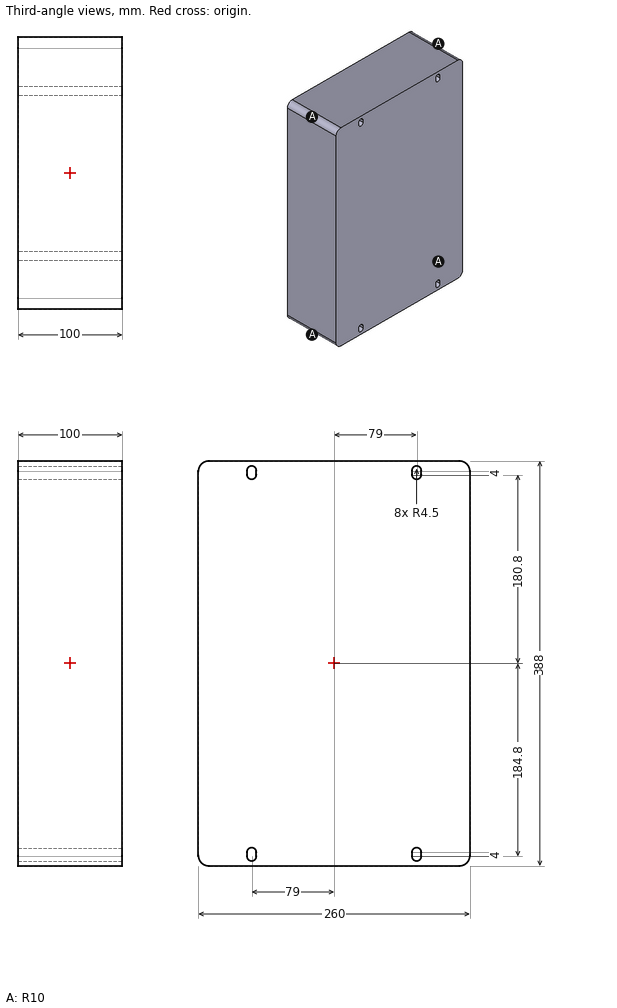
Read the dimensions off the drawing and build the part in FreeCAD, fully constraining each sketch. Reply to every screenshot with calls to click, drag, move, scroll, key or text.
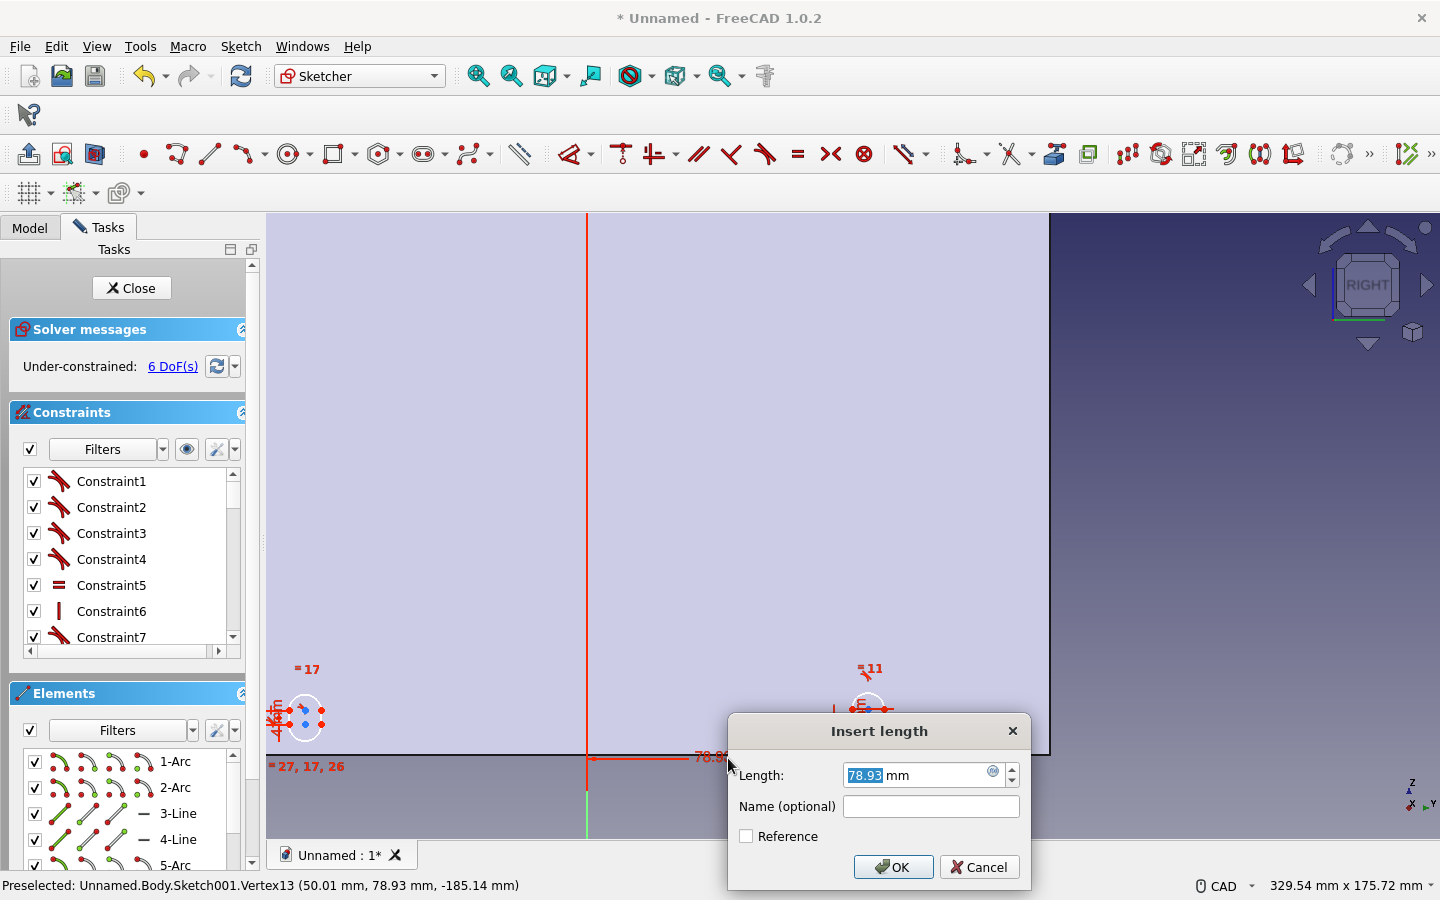
text(79)
key(Return)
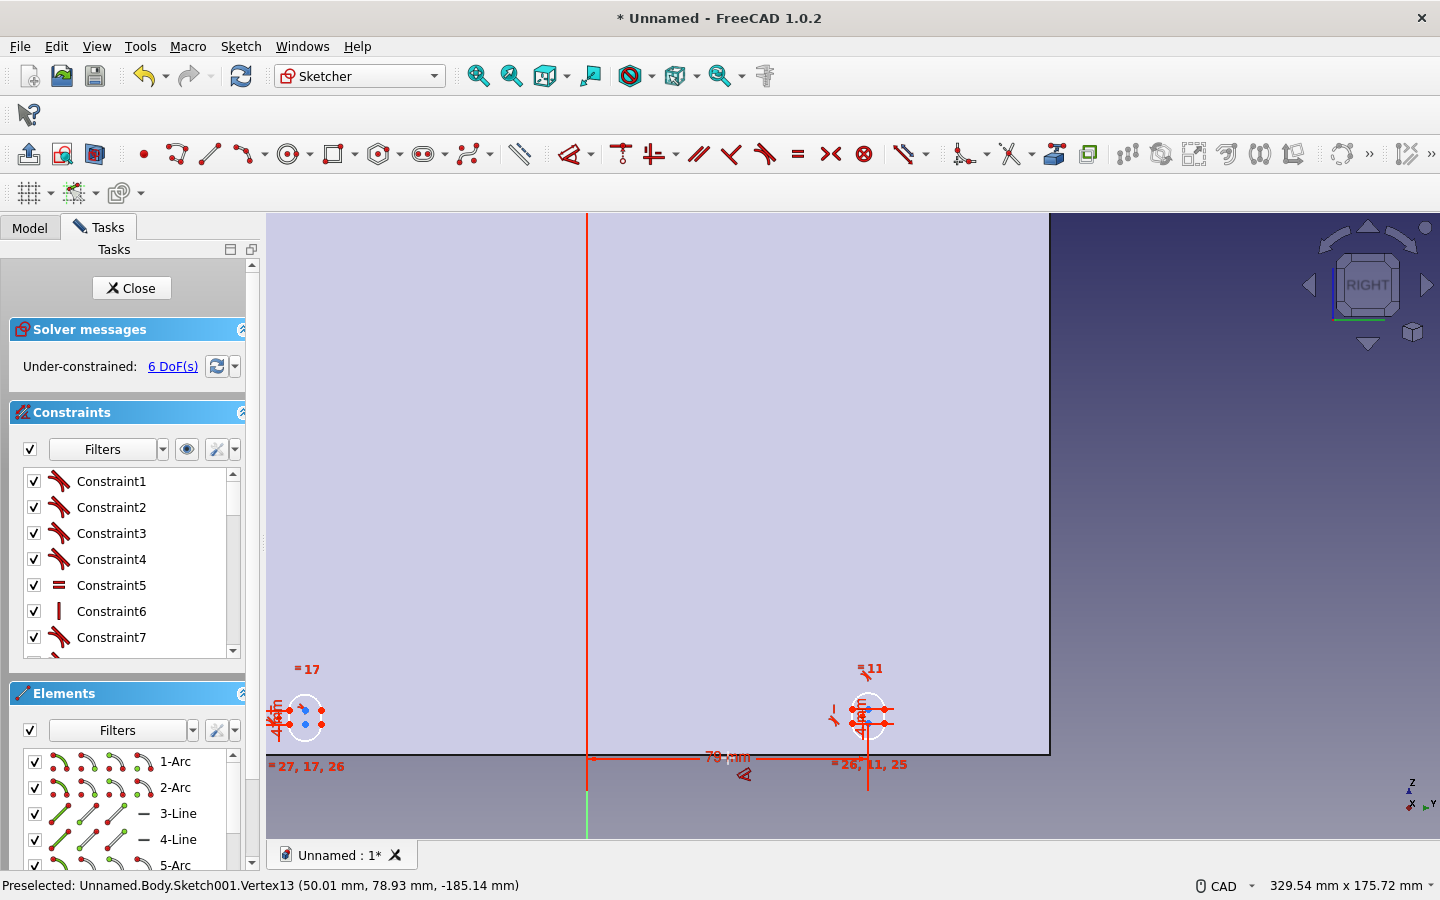
click(305, 725)
click(446, 759)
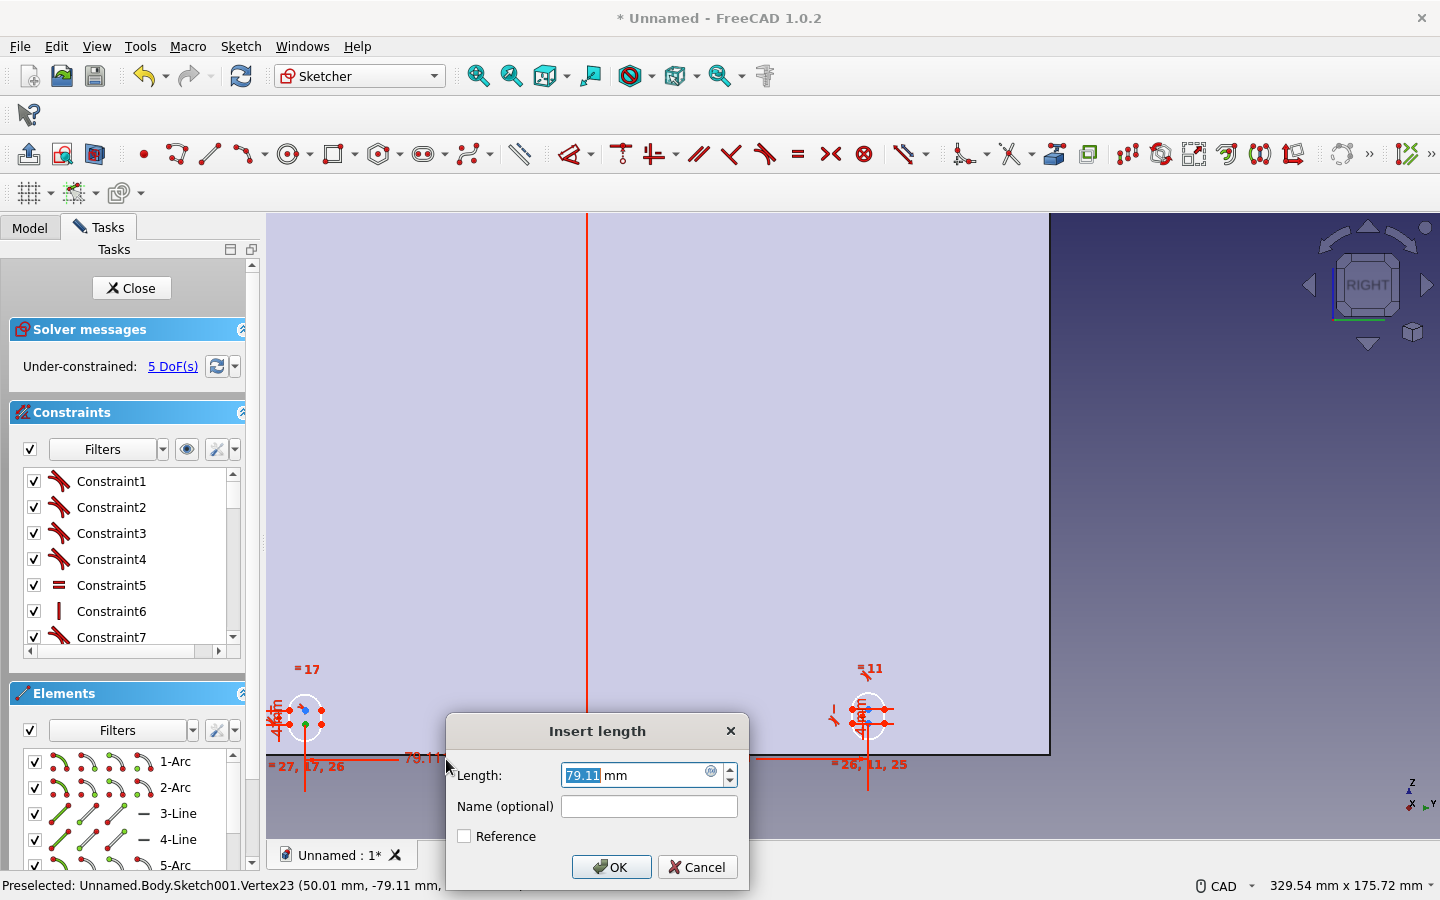
text(79)
key(Return)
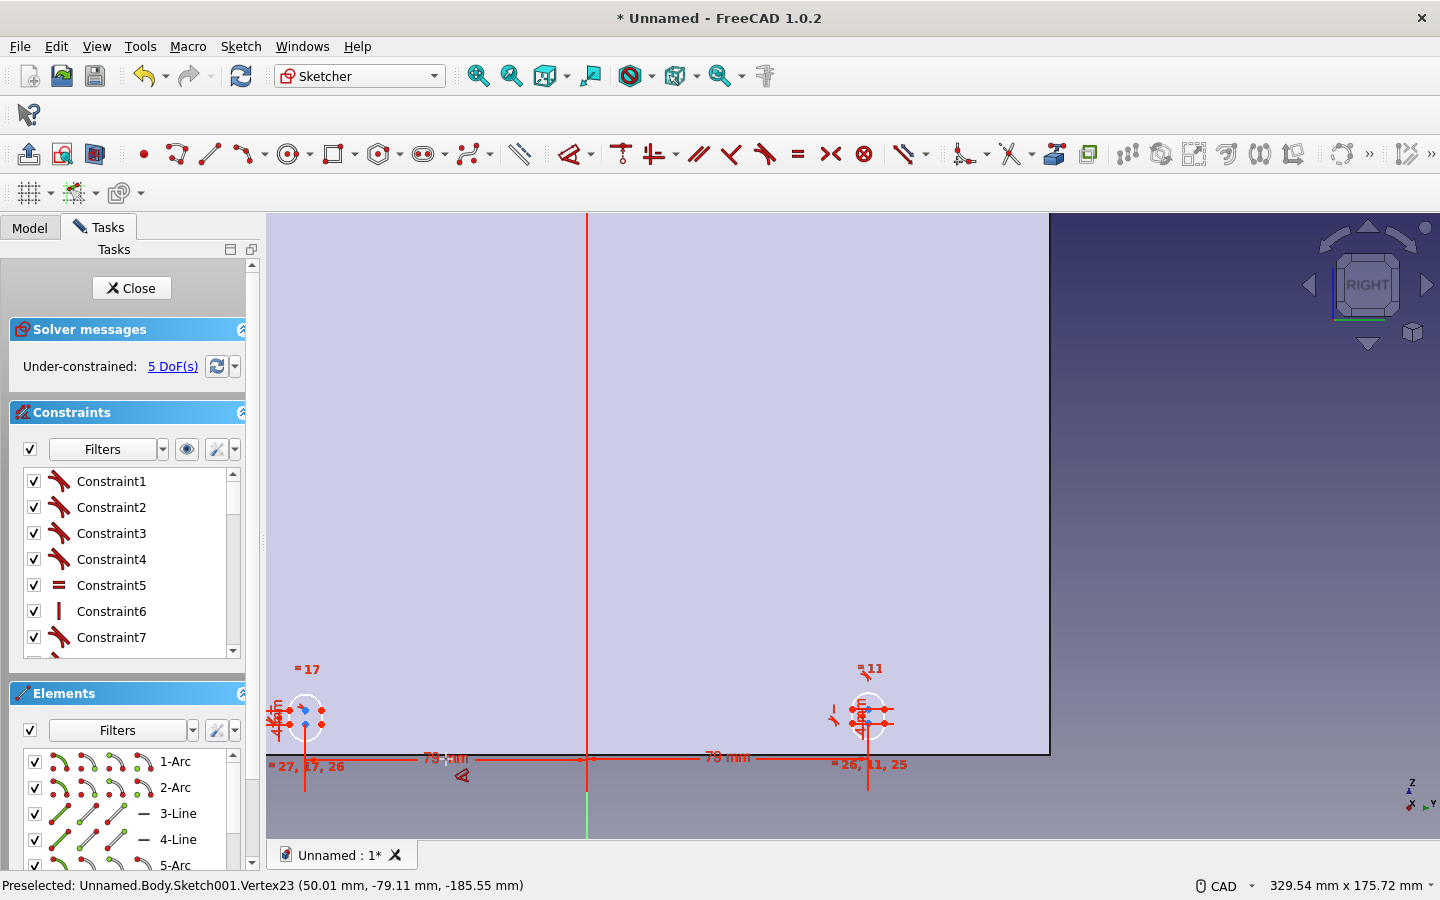
scroll(870, 725, down, 6)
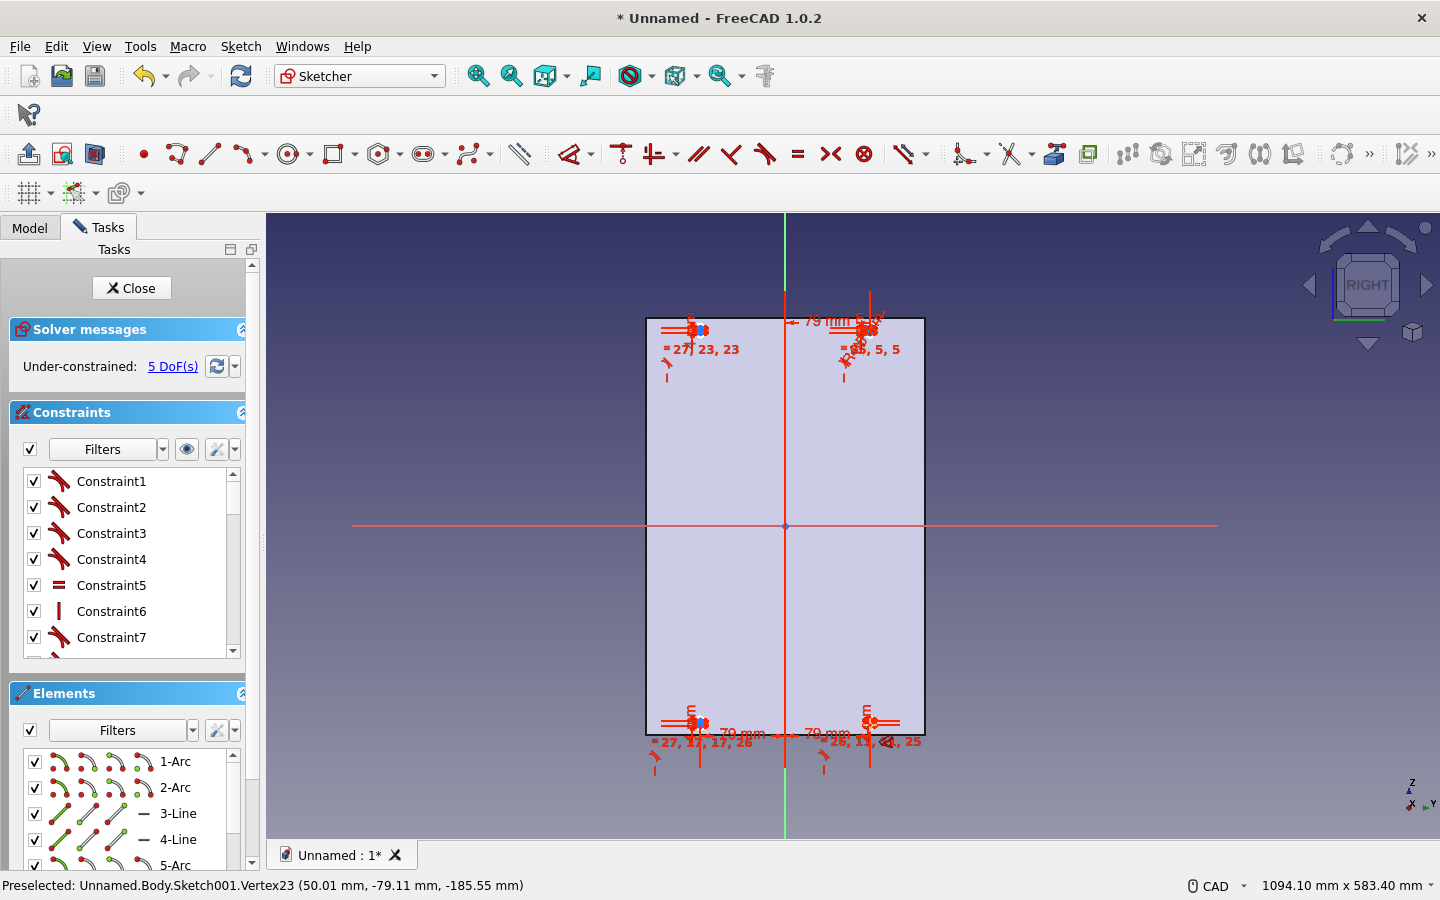
scroll(700, 333, up, 6)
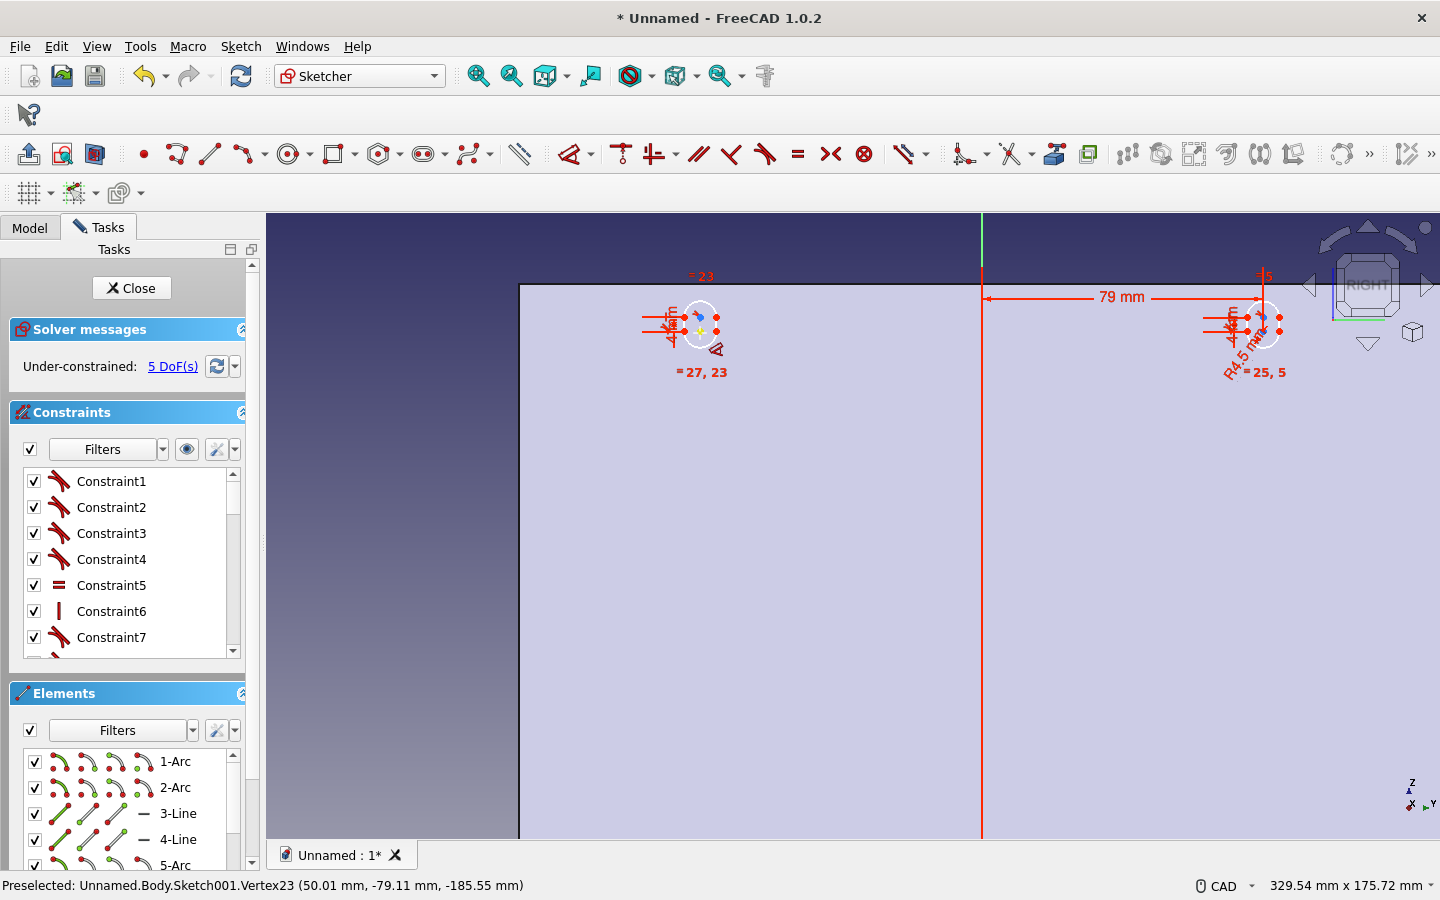
click(700, 332)
click(841, 298)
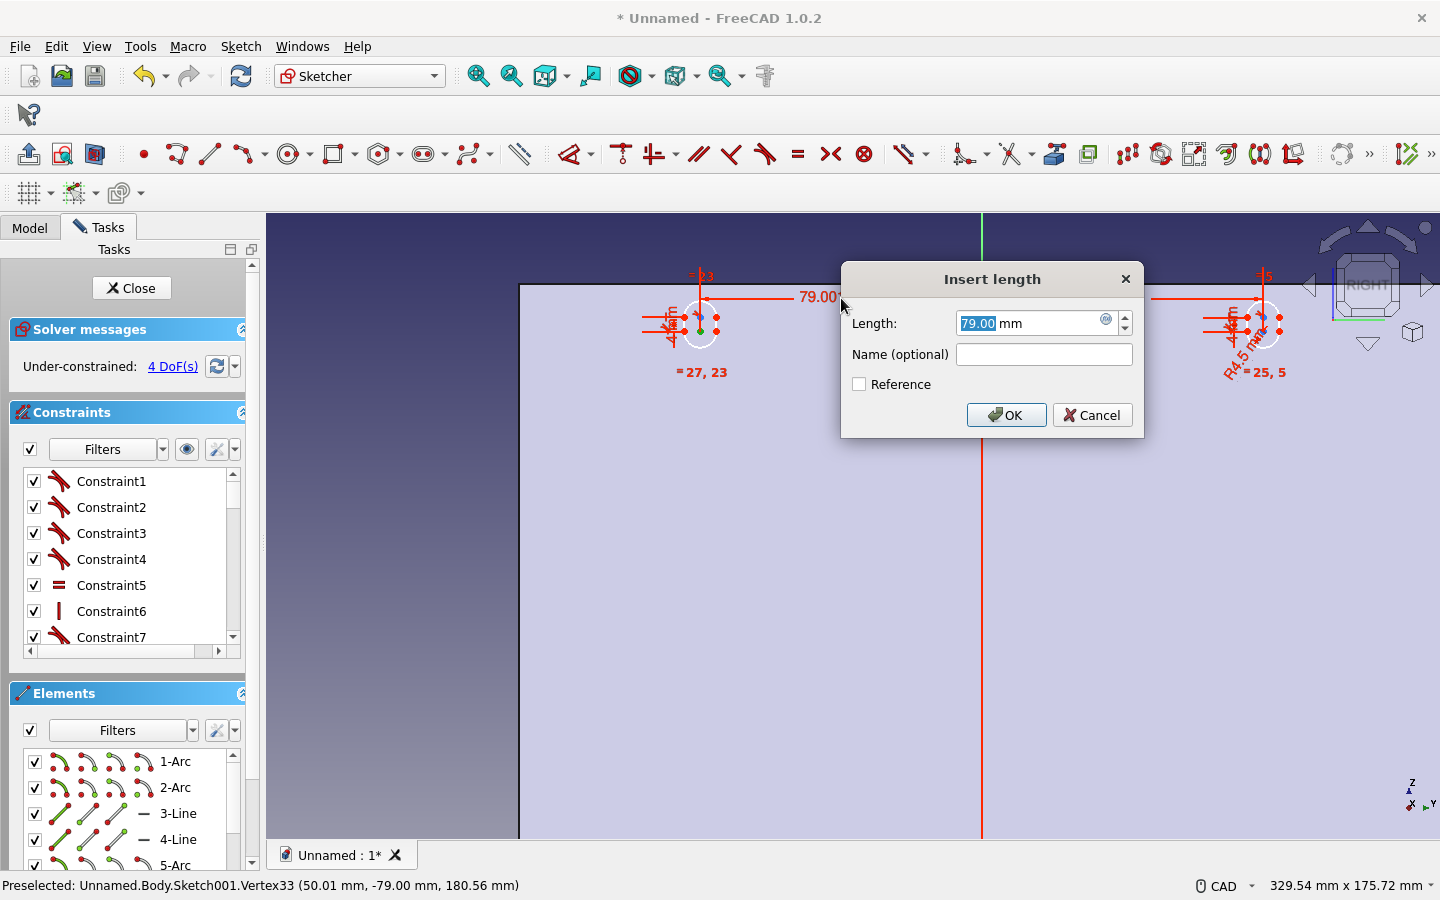
text(79)
key(Return)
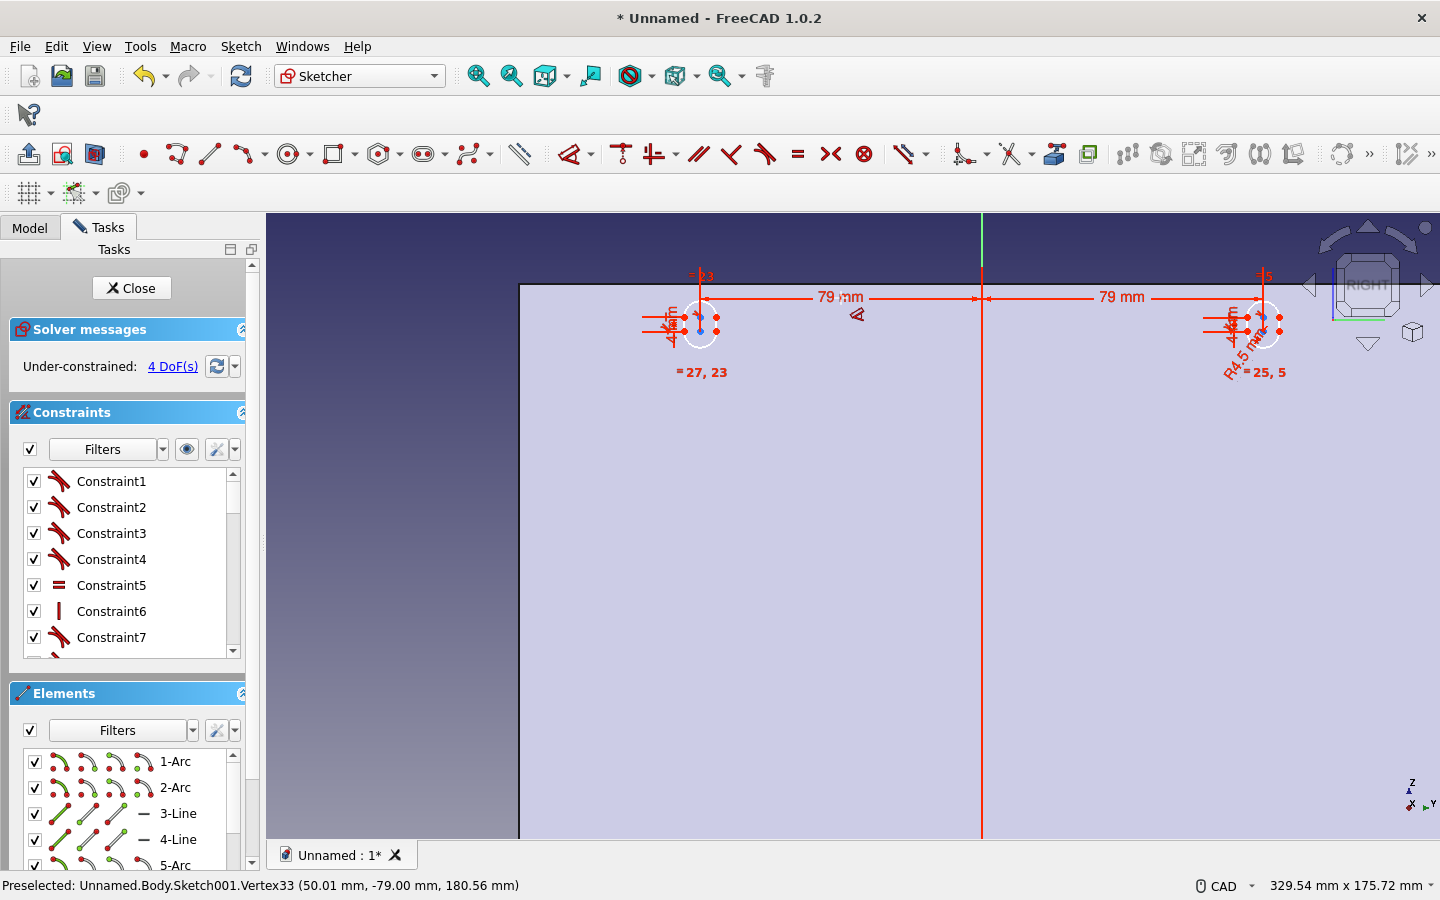
click(1247, 332)
click(948, 571)